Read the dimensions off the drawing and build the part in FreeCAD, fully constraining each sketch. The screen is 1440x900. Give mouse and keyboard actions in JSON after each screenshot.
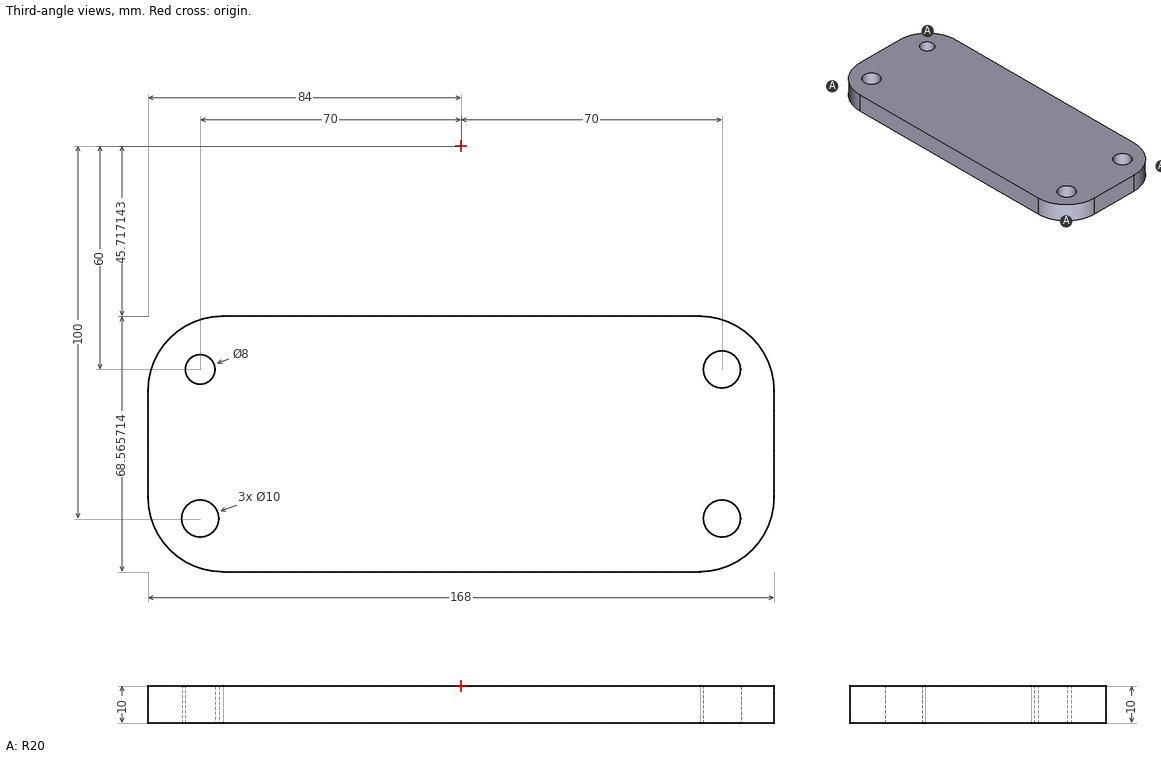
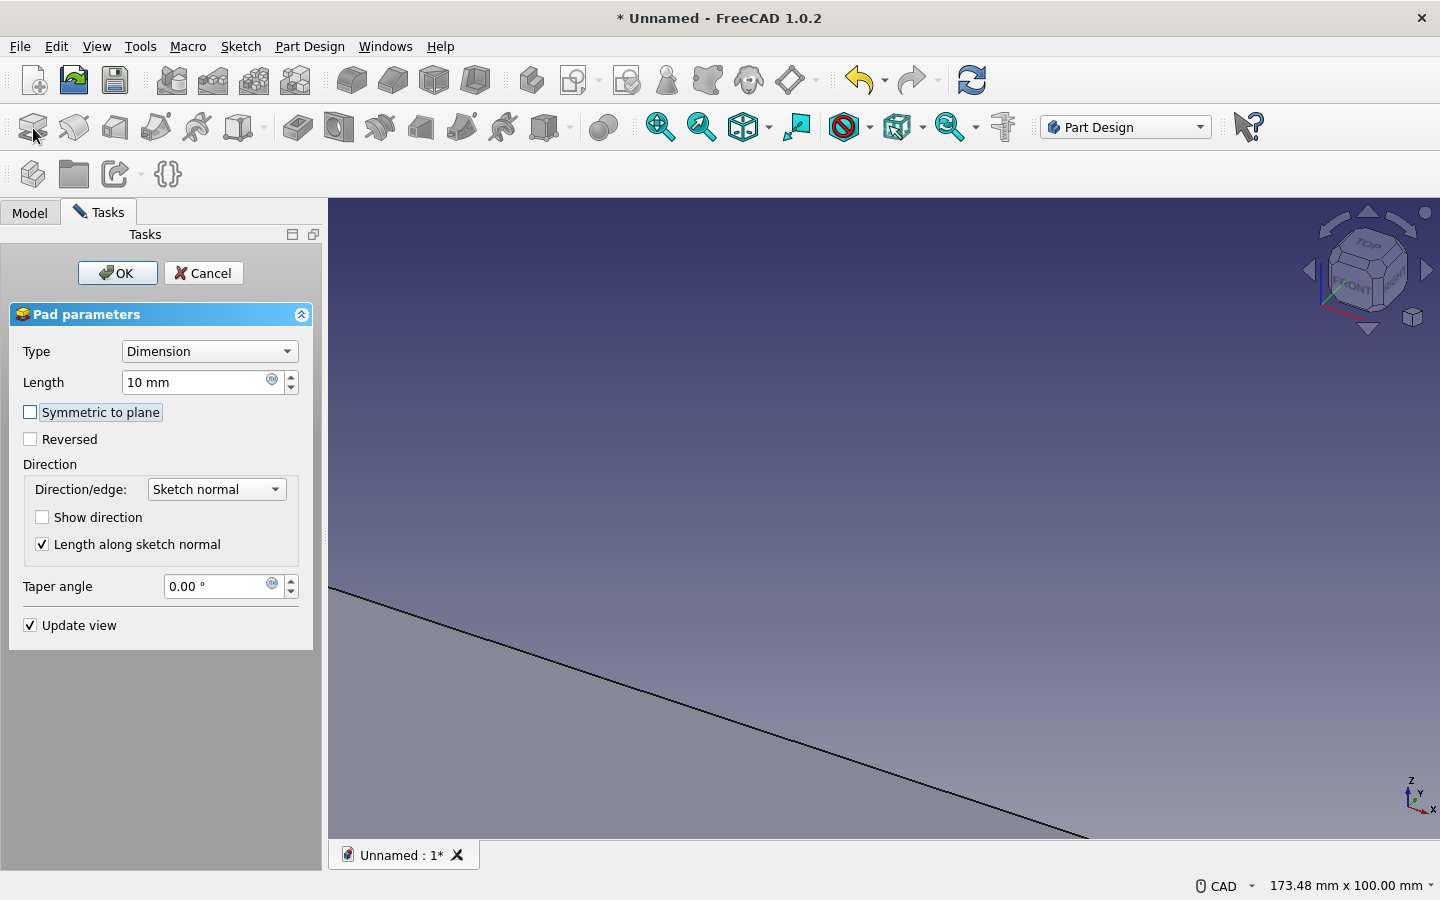
{"action": "left_click", "coordinate": [31, 439]}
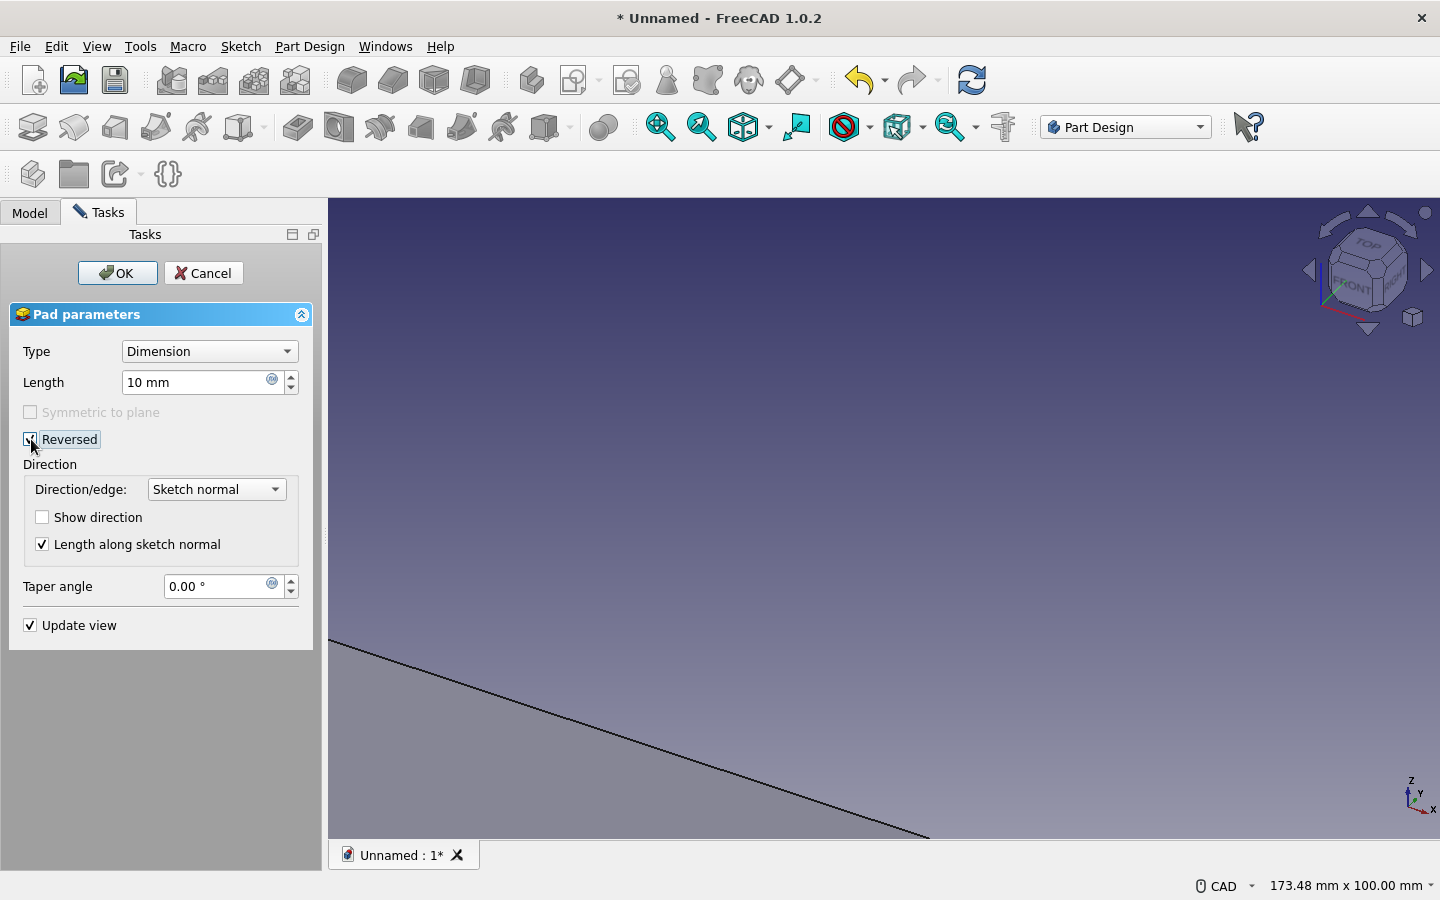
{"action": "left_click", "coordinate": [118, 273]}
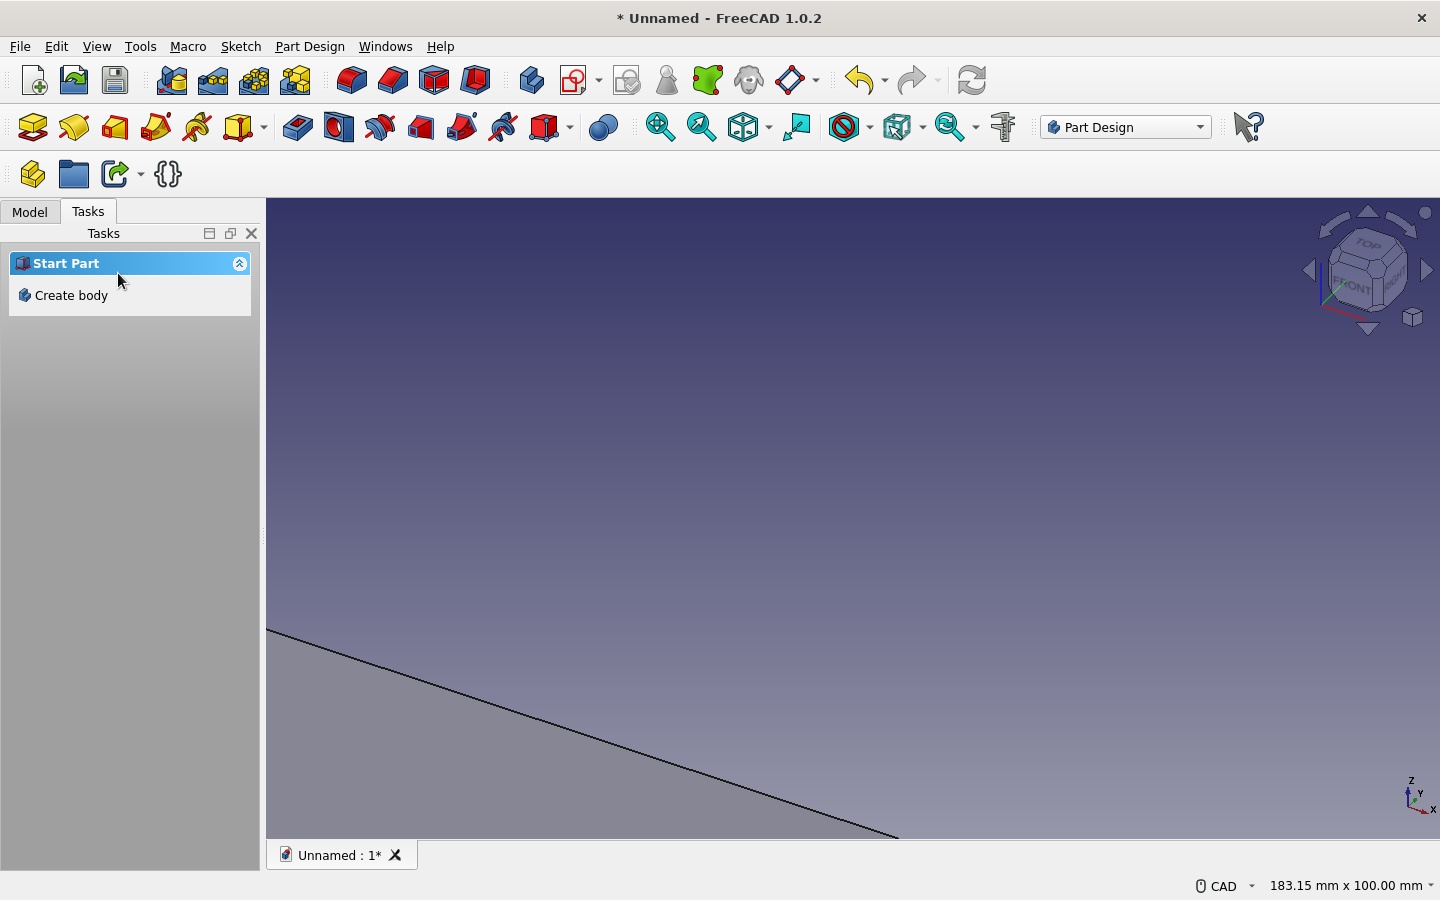
{"action": "left_click", "coordinate": [661, 128]}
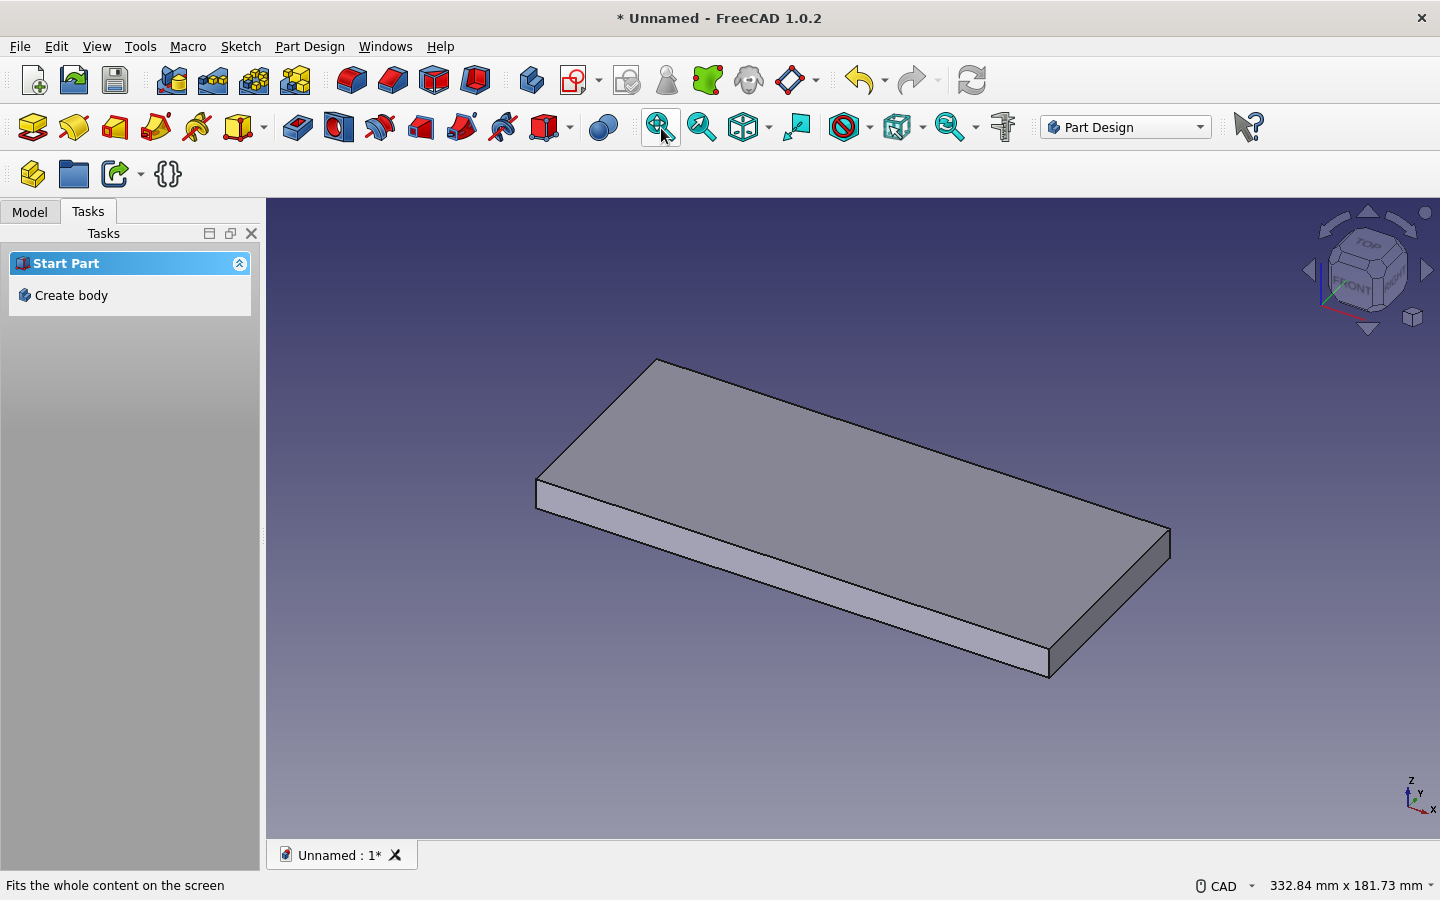
{"action": "left_click", "coordinate": [1000, 552]}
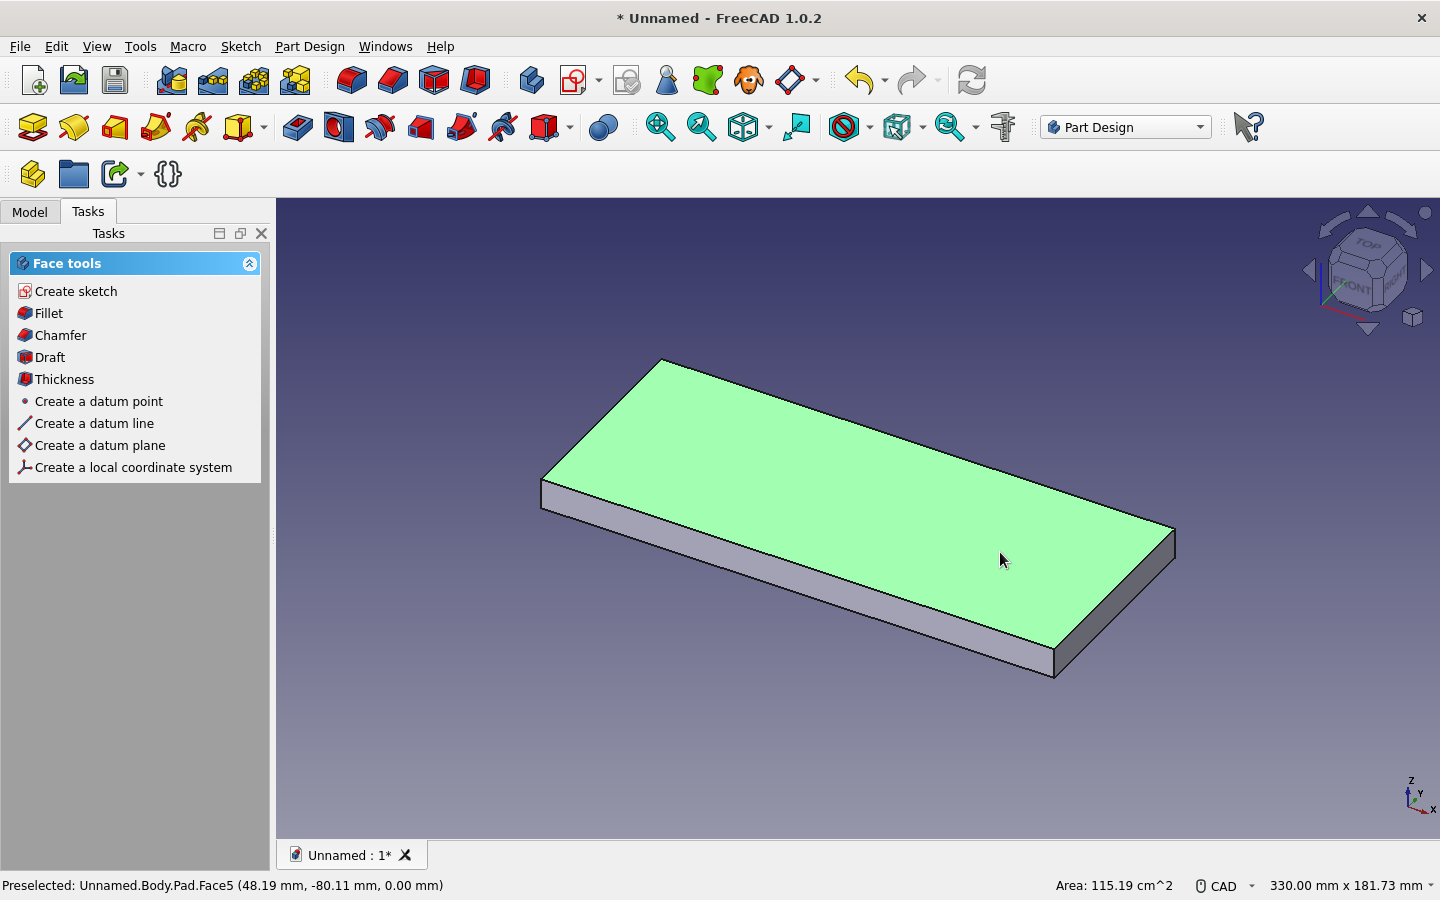
{"action": "left_click", "coordinate": [572, 80]}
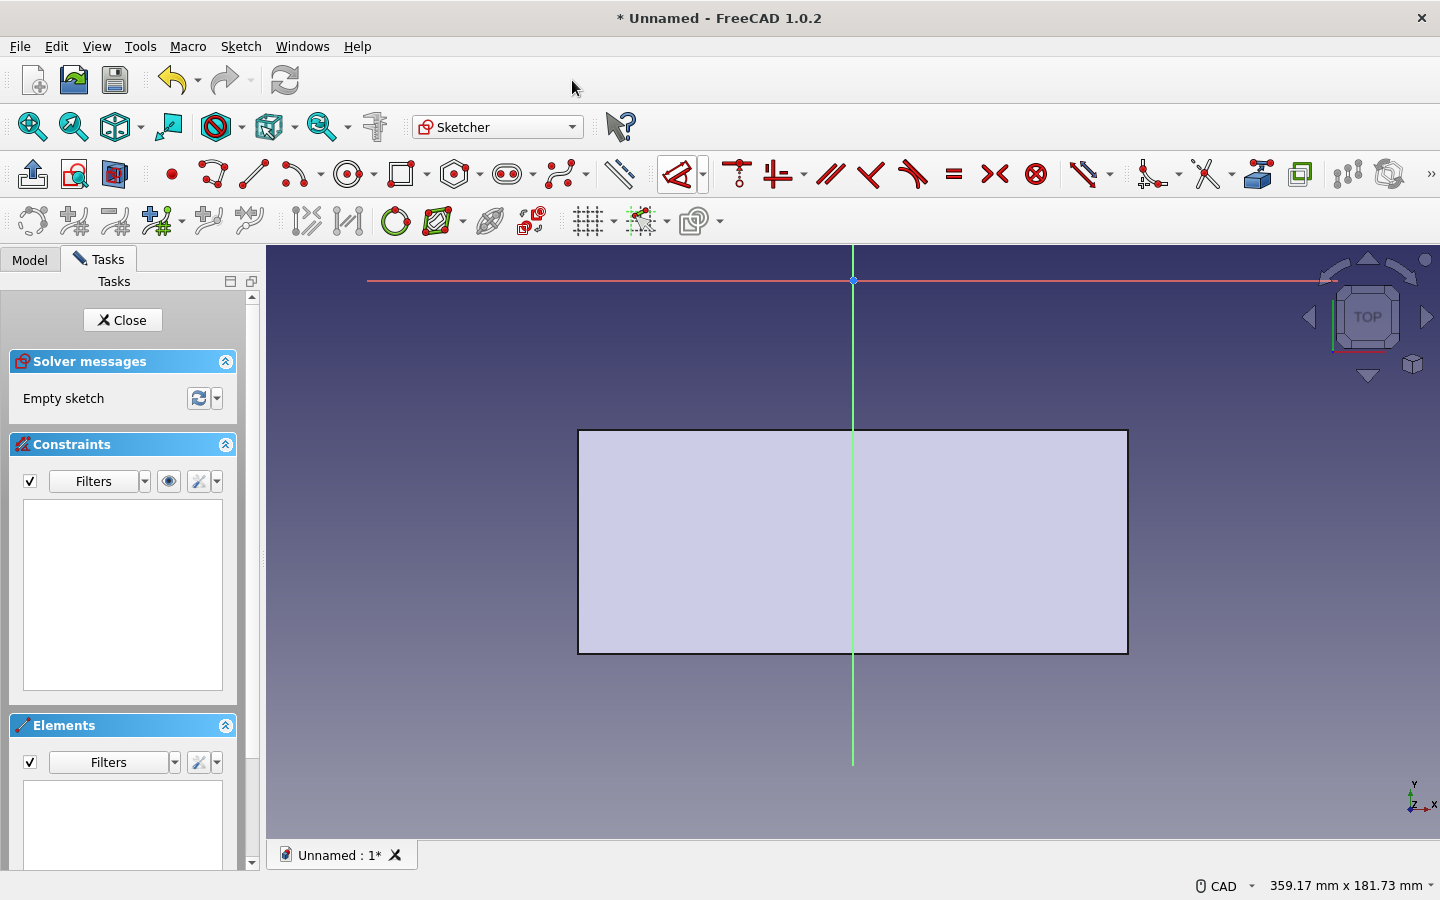
{"action": "scroll", "coordinate": [475, 811], "scroll_direction": "down", "scroll_amount": 1}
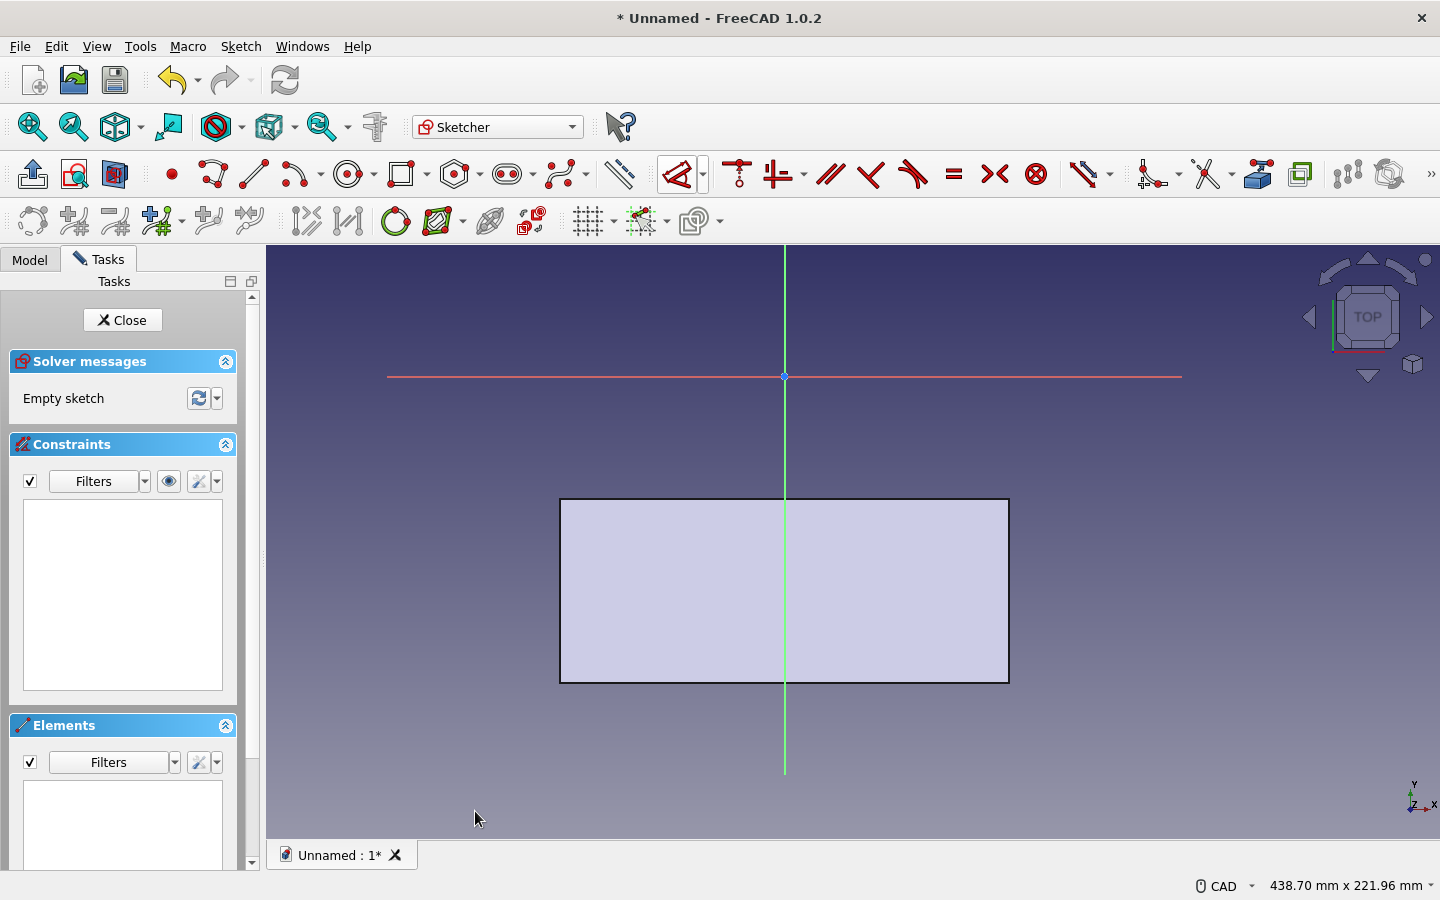
{"action": "scroll", "coordinate": [785, 467], "scroll_direction": "up", "scroll_amount": 2}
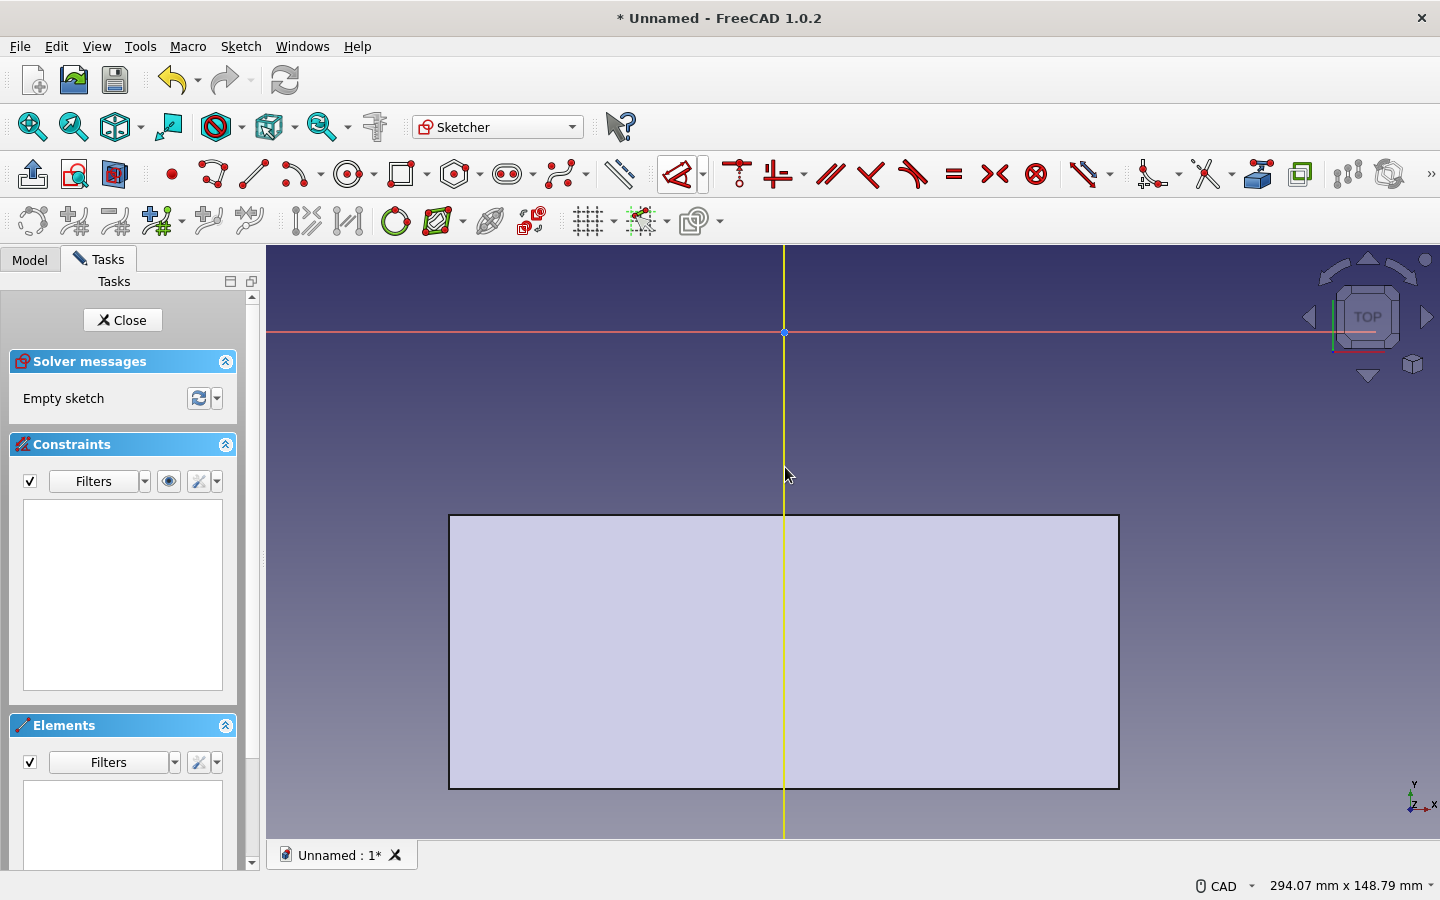
{"action": "left_click", "coordinate": [348, 174]}